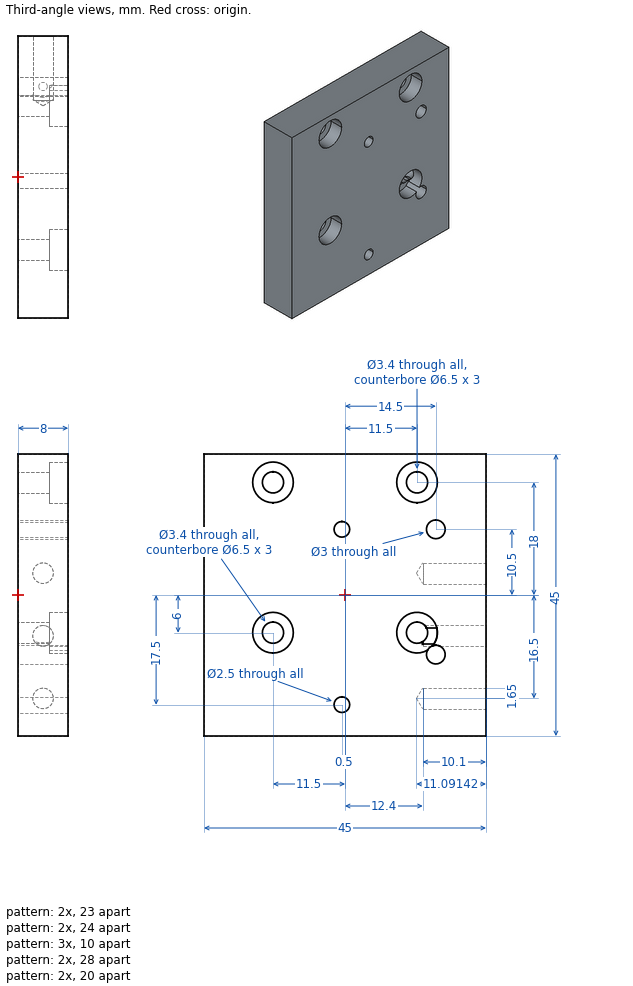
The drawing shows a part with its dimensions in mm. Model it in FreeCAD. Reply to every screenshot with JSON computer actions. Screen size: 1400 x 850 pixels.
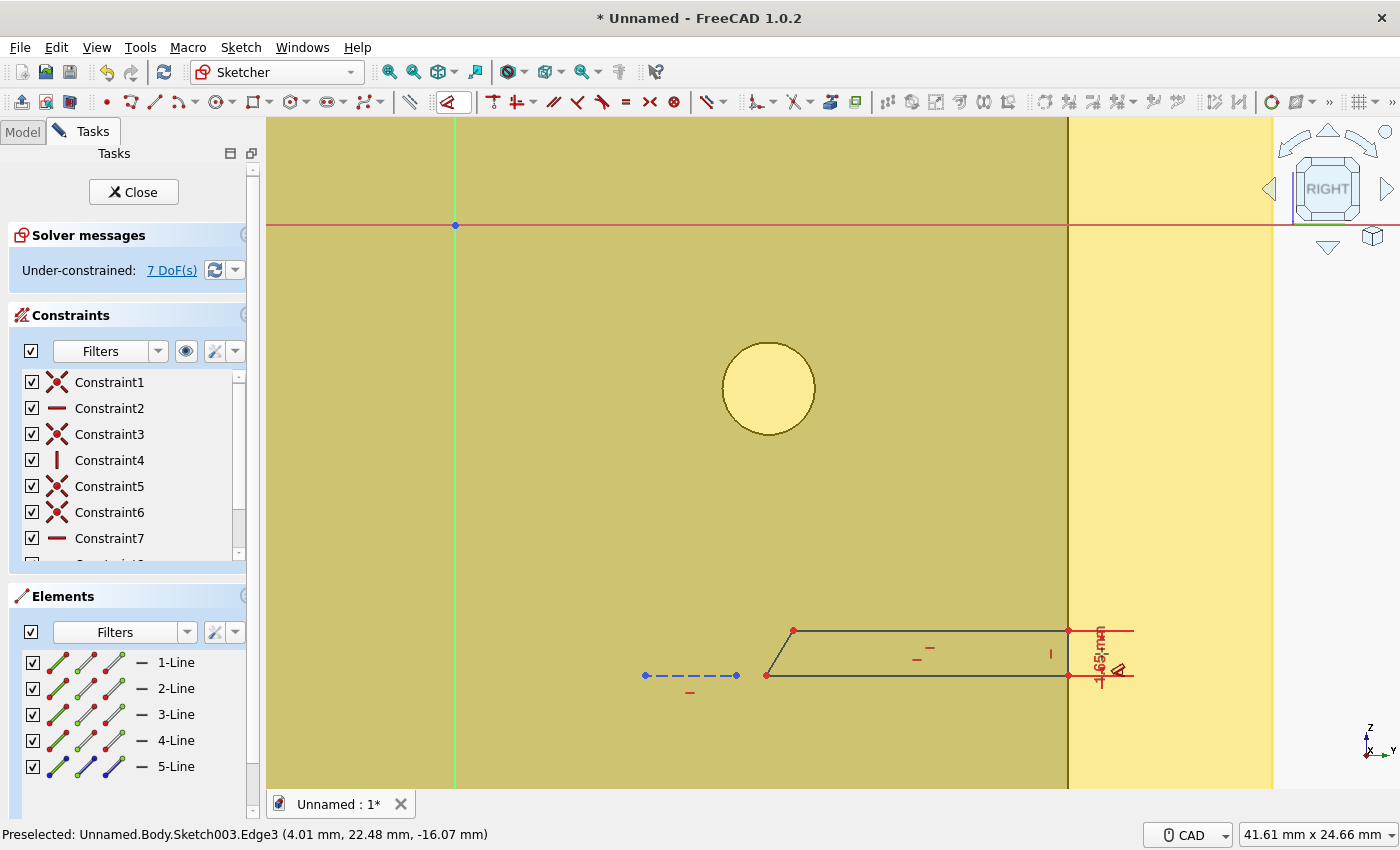
{"action": "left_click", "coordinate": [986, 631]}
{"action": "left_click", "coordinate": [931, 597]}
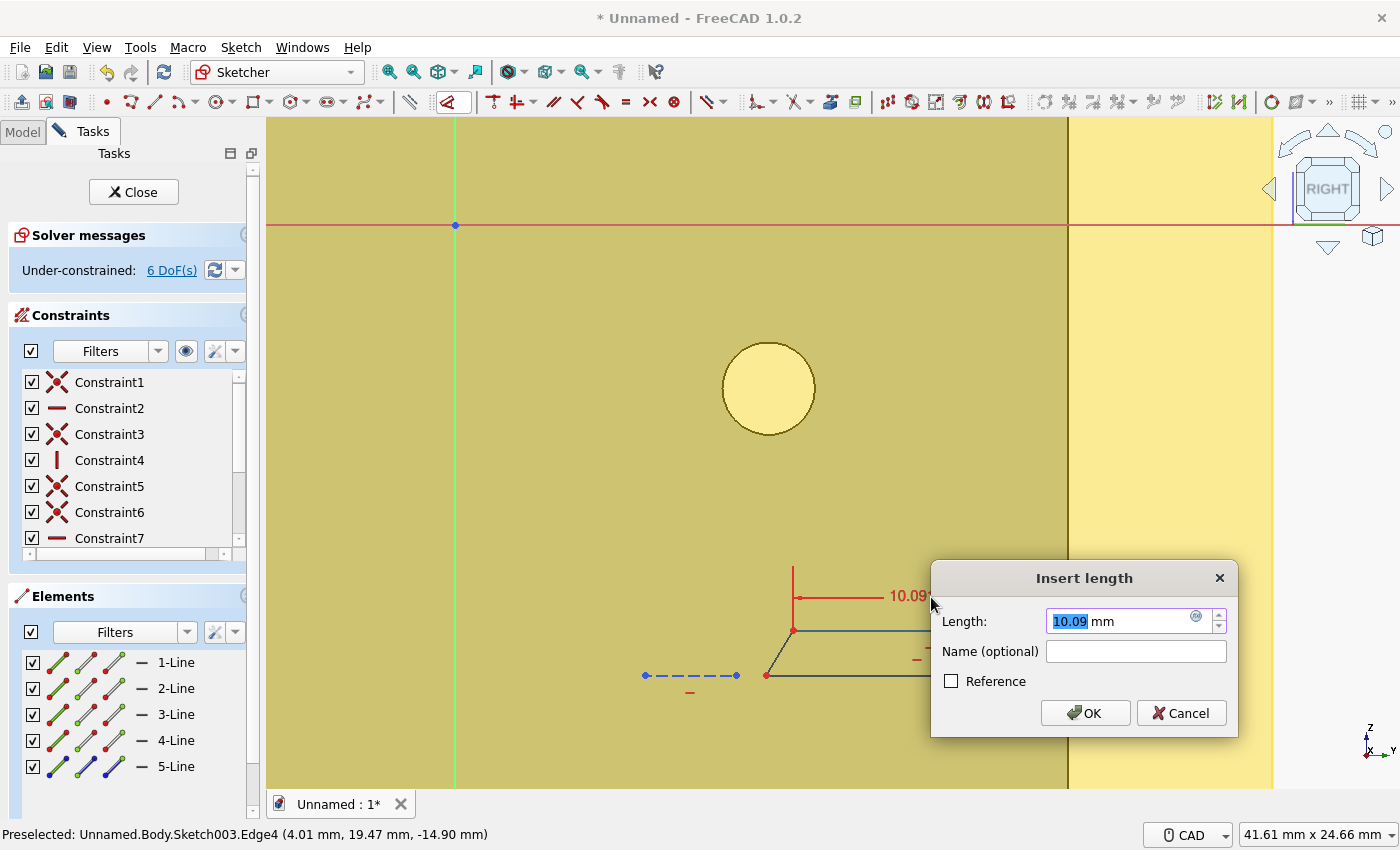
{"action": "type", "text": "10.1"}
{"action": "key", "text": "Return"}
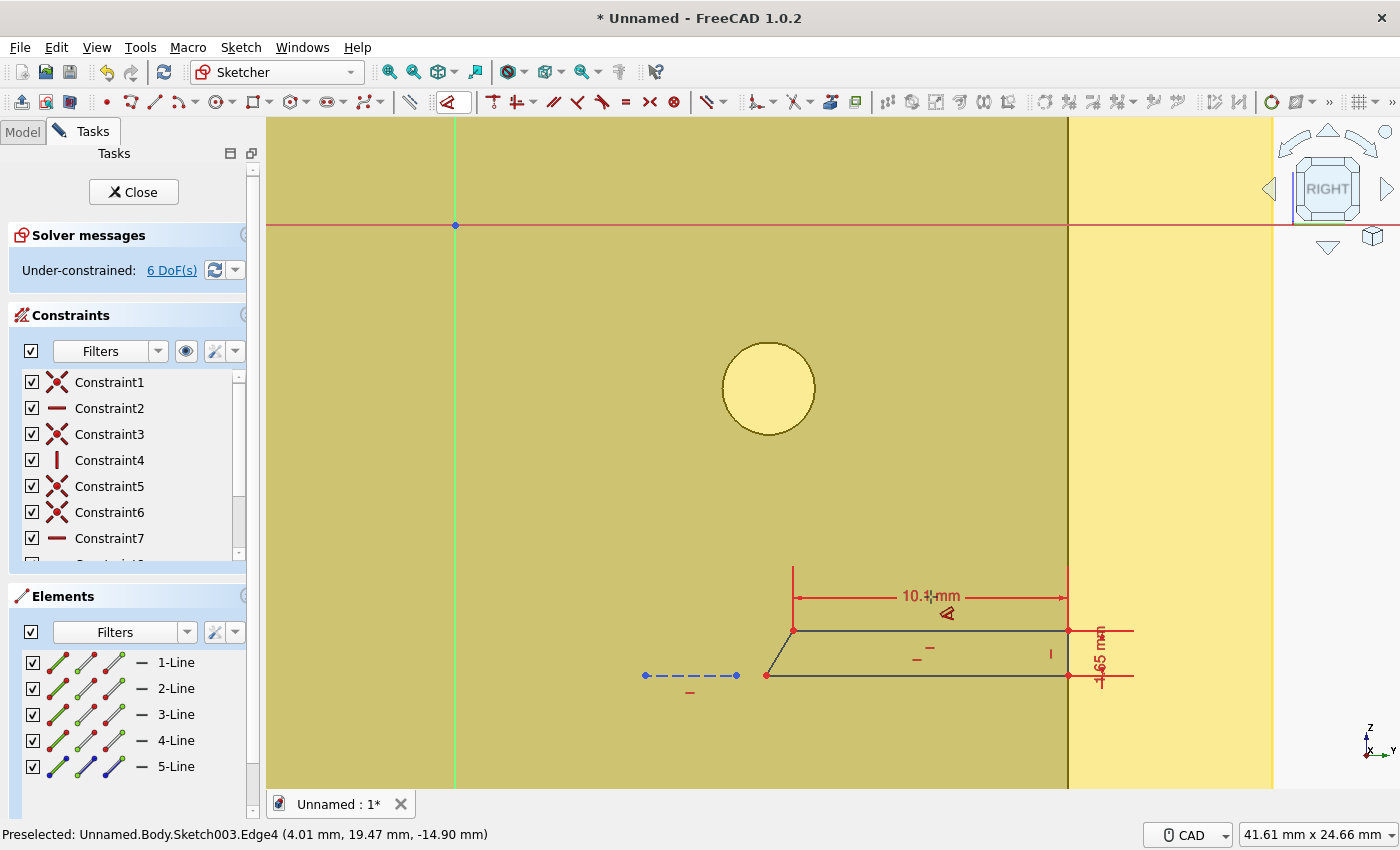
{"action": "left_click", "coordinate": [793, 631]}
{"action": "left_click", "coordinate": [624, 191]}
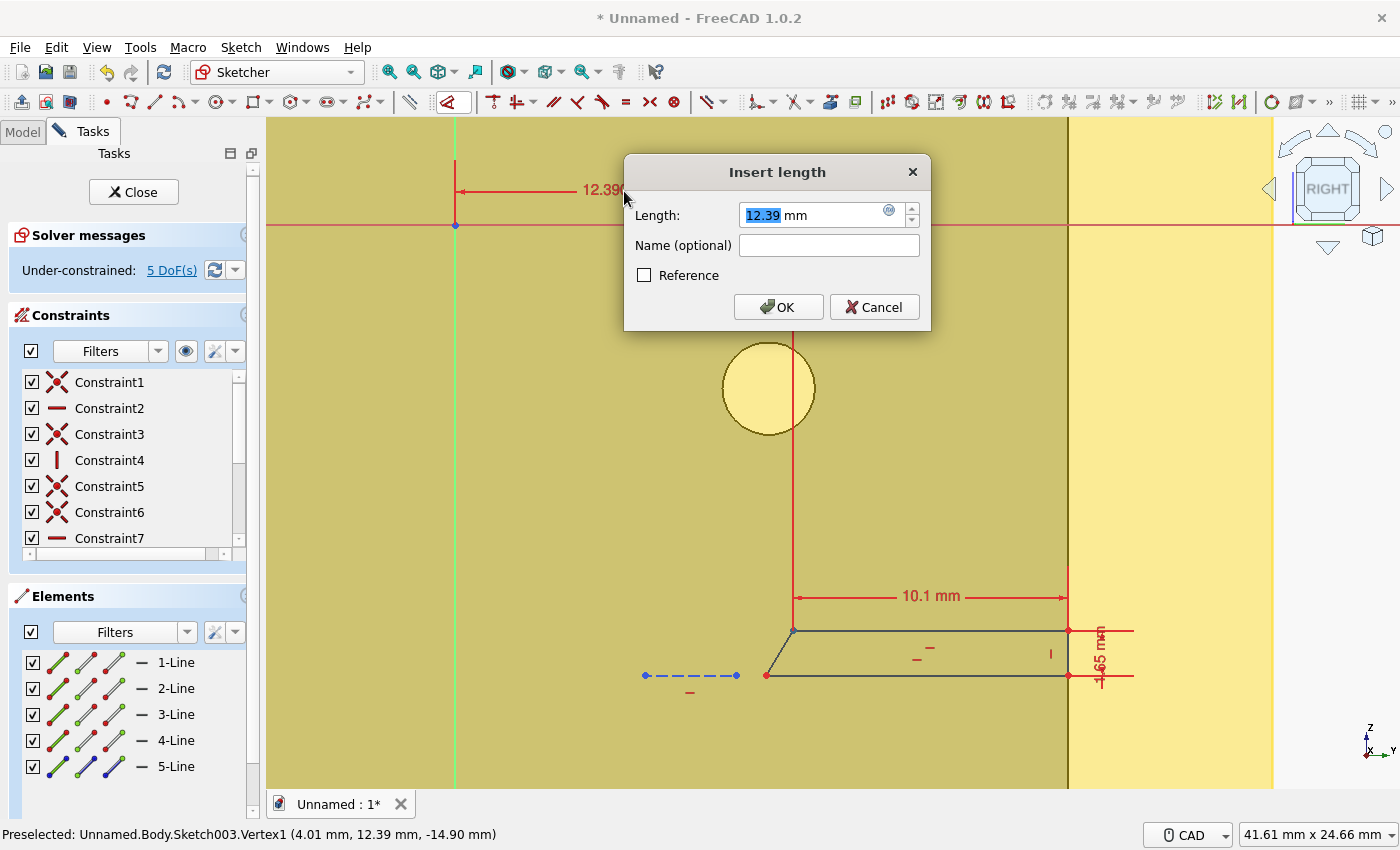
{"action": "type", "text": "12.4"}
{"action": "key", "text": "Return"}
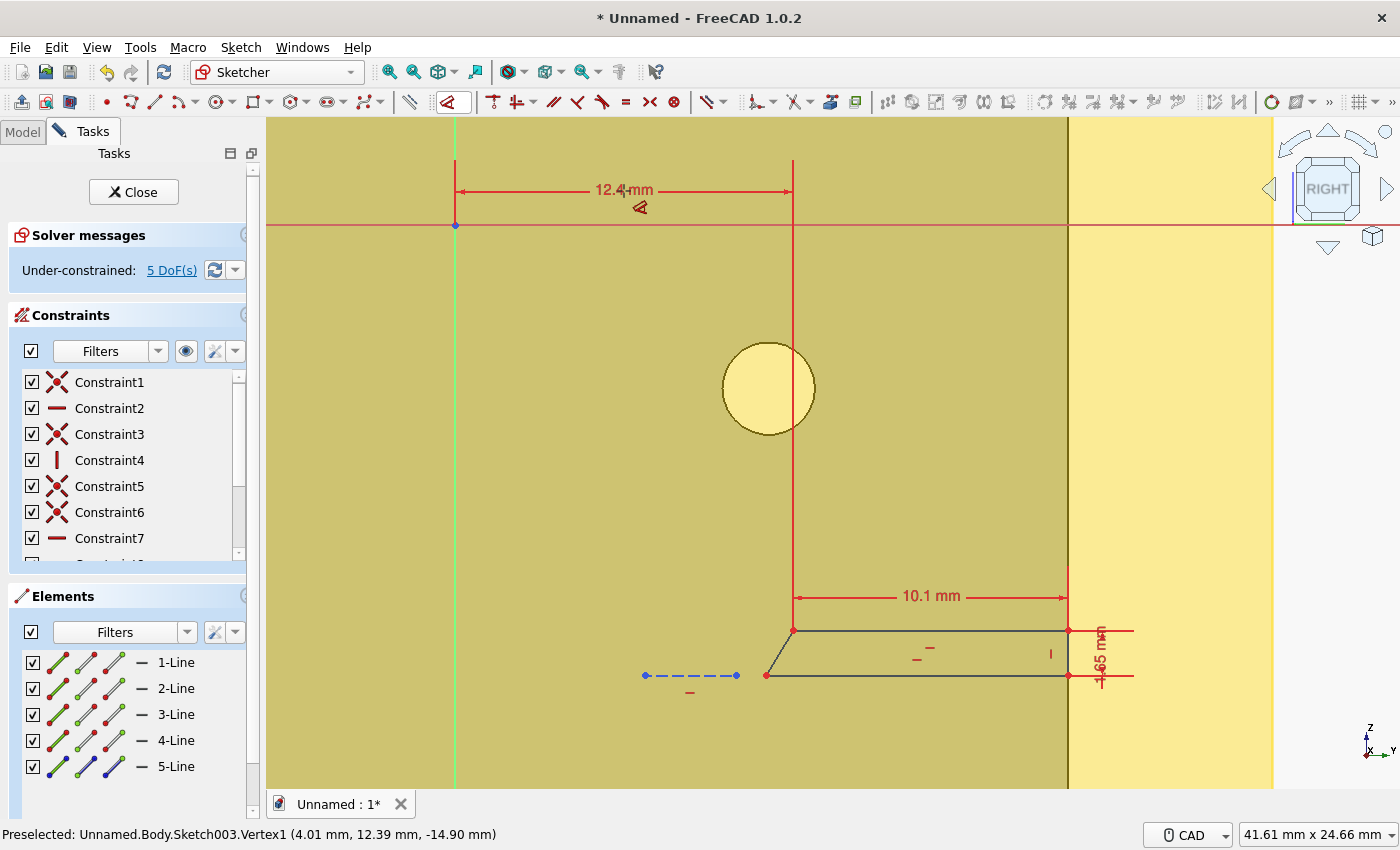
{"action": "left_click", "coordinate": [766, 676]}
{"action": "left_click", "coordinate": [421, 451]}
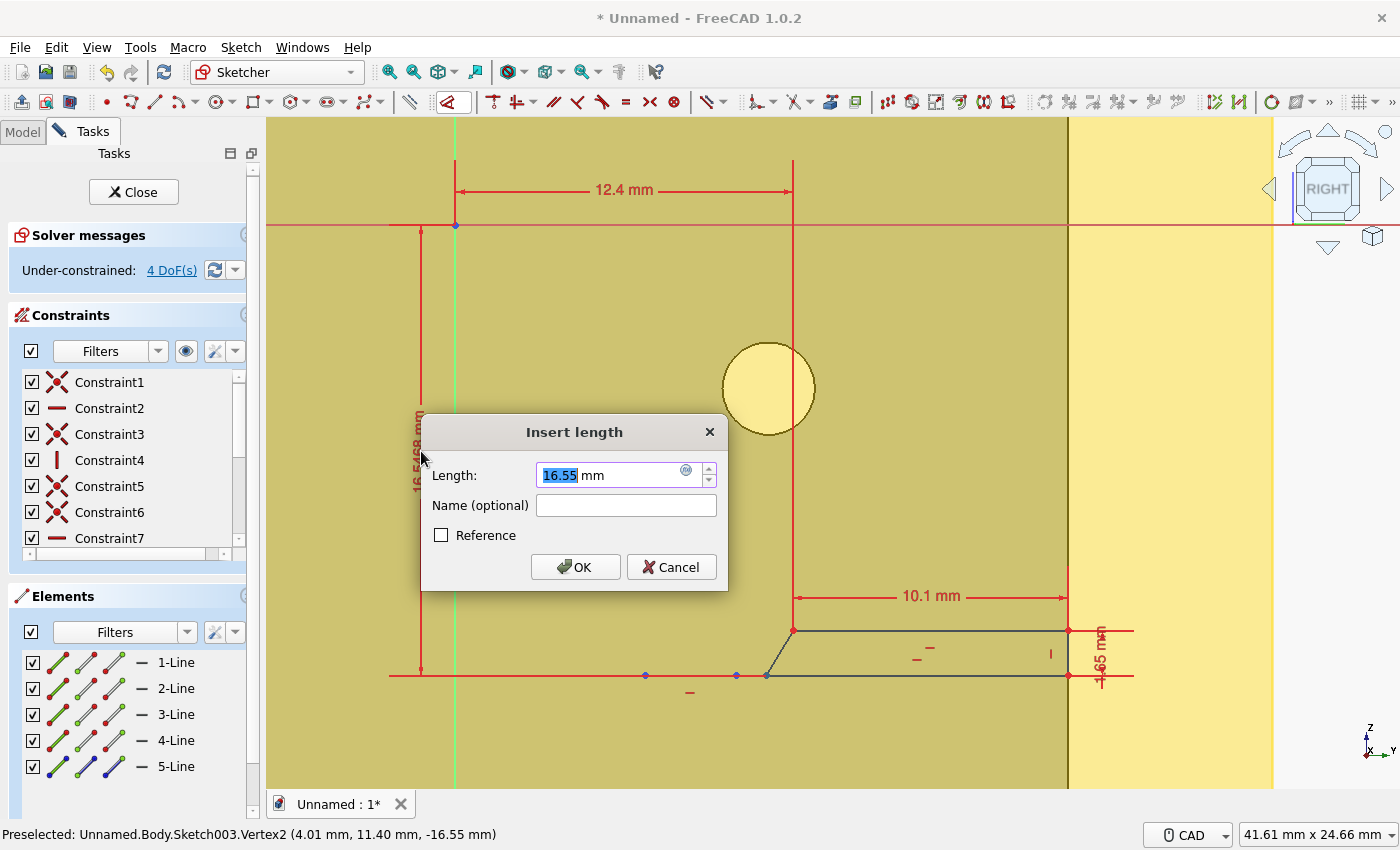
{"action": "type", "text": "16.5"}
{"action": "key", "text": "Return"}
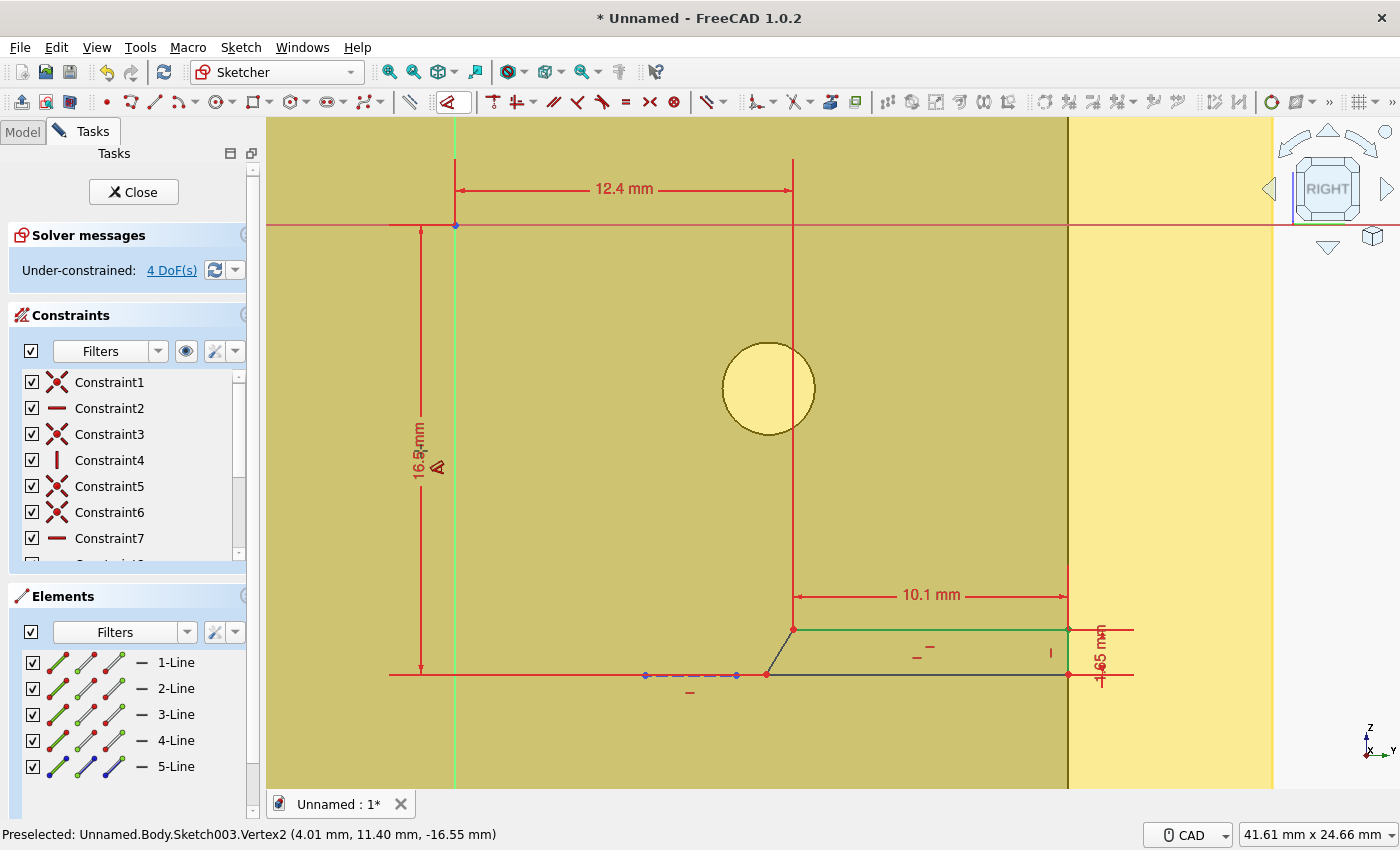
{"action": "left_click", "coordinate": [736, 676]}
{"action": "left_click", "coordinate": [421, 347]}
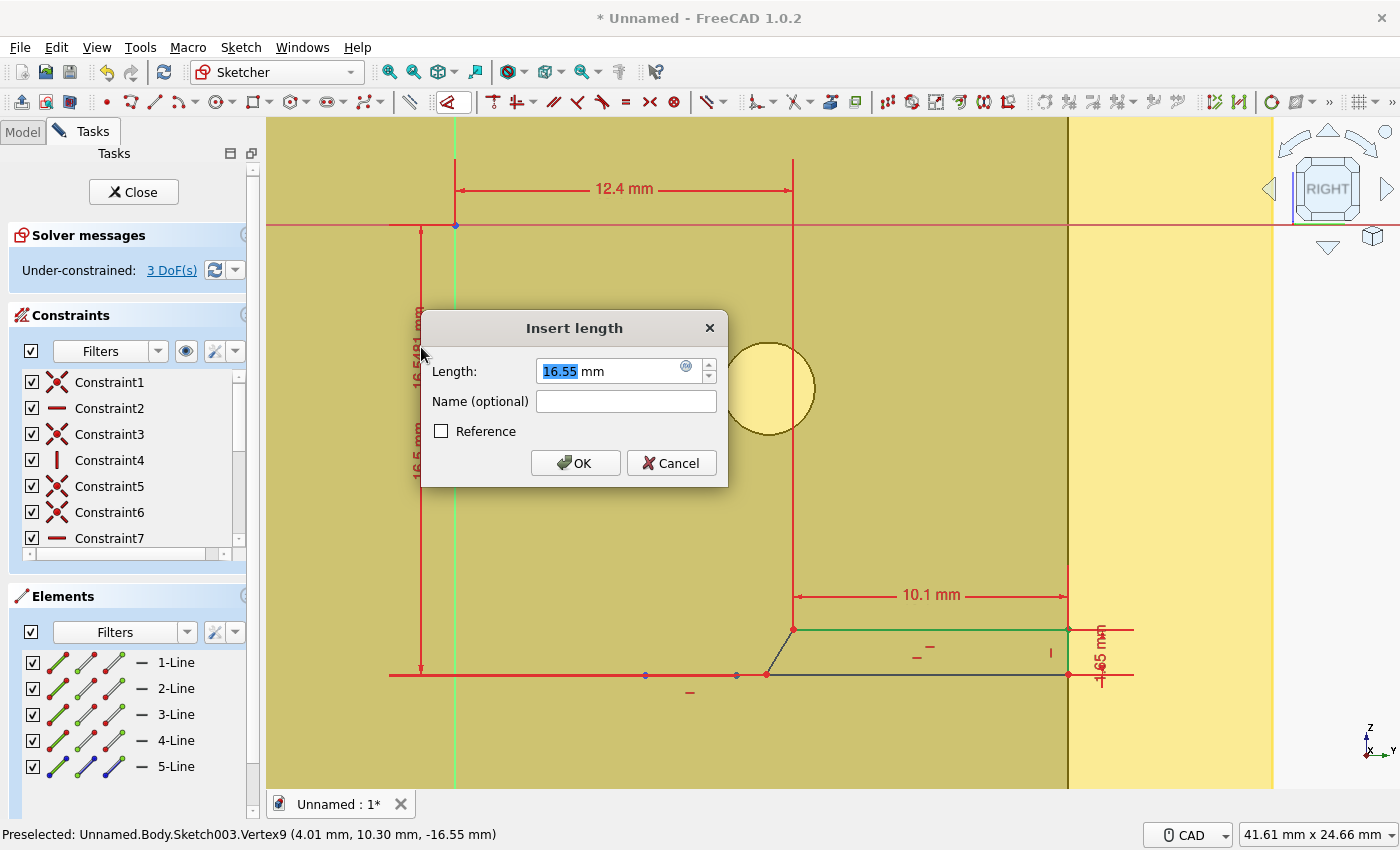
{"action": "type", "text": "16.5"}
{"action": "key", "text": "Return"}